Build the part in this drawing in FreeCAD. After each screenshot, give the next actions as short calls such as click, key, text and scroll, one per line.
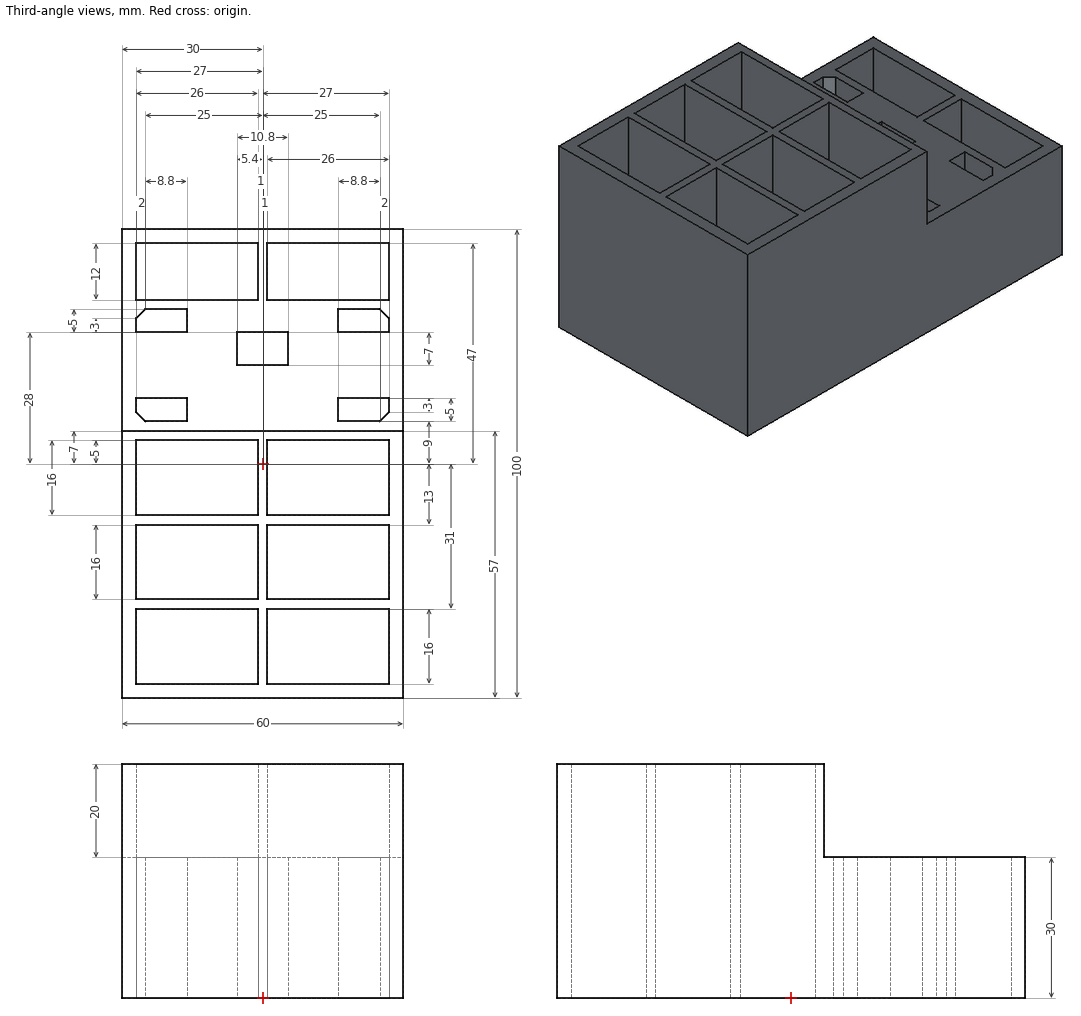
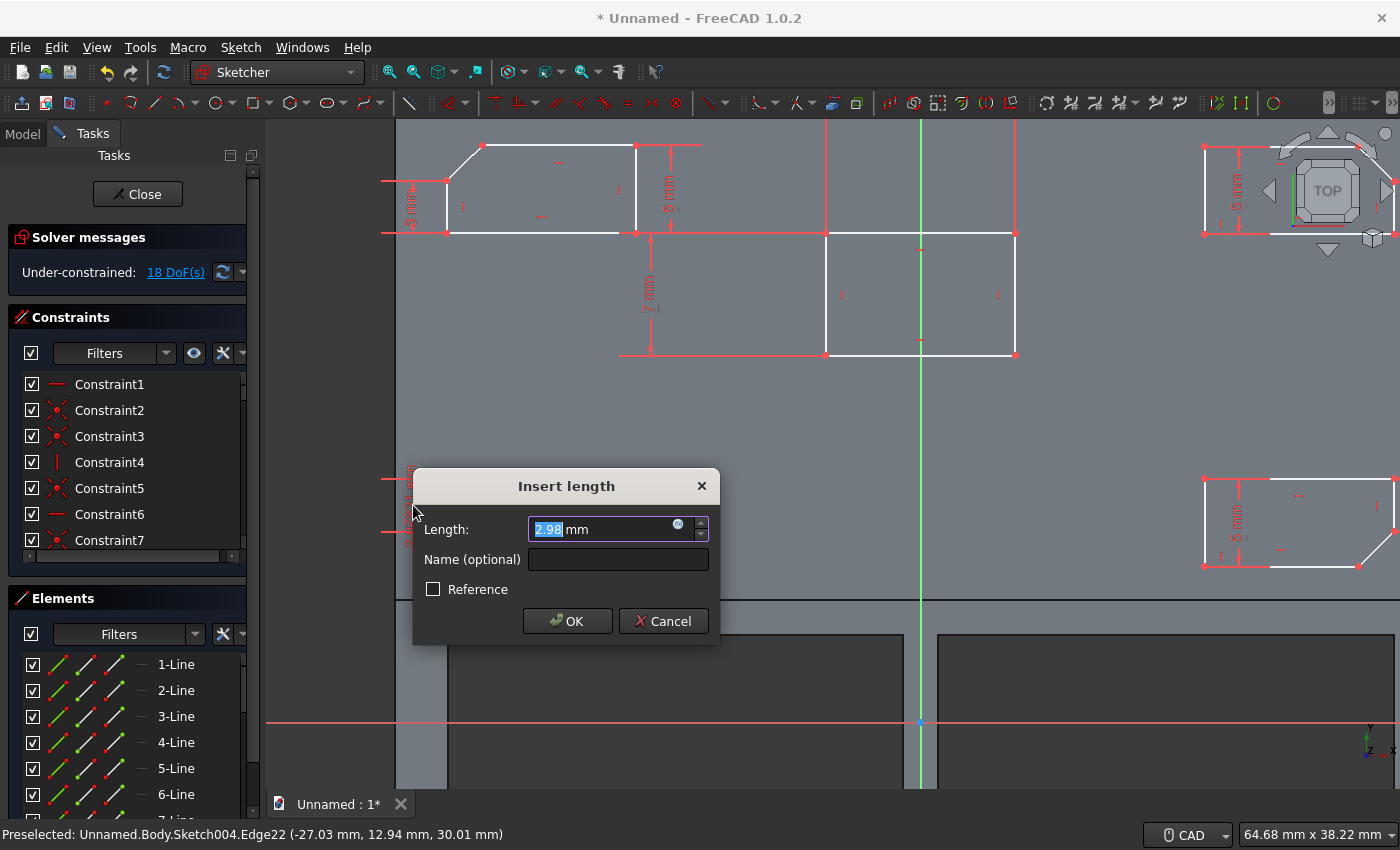
text(3)
key(Return)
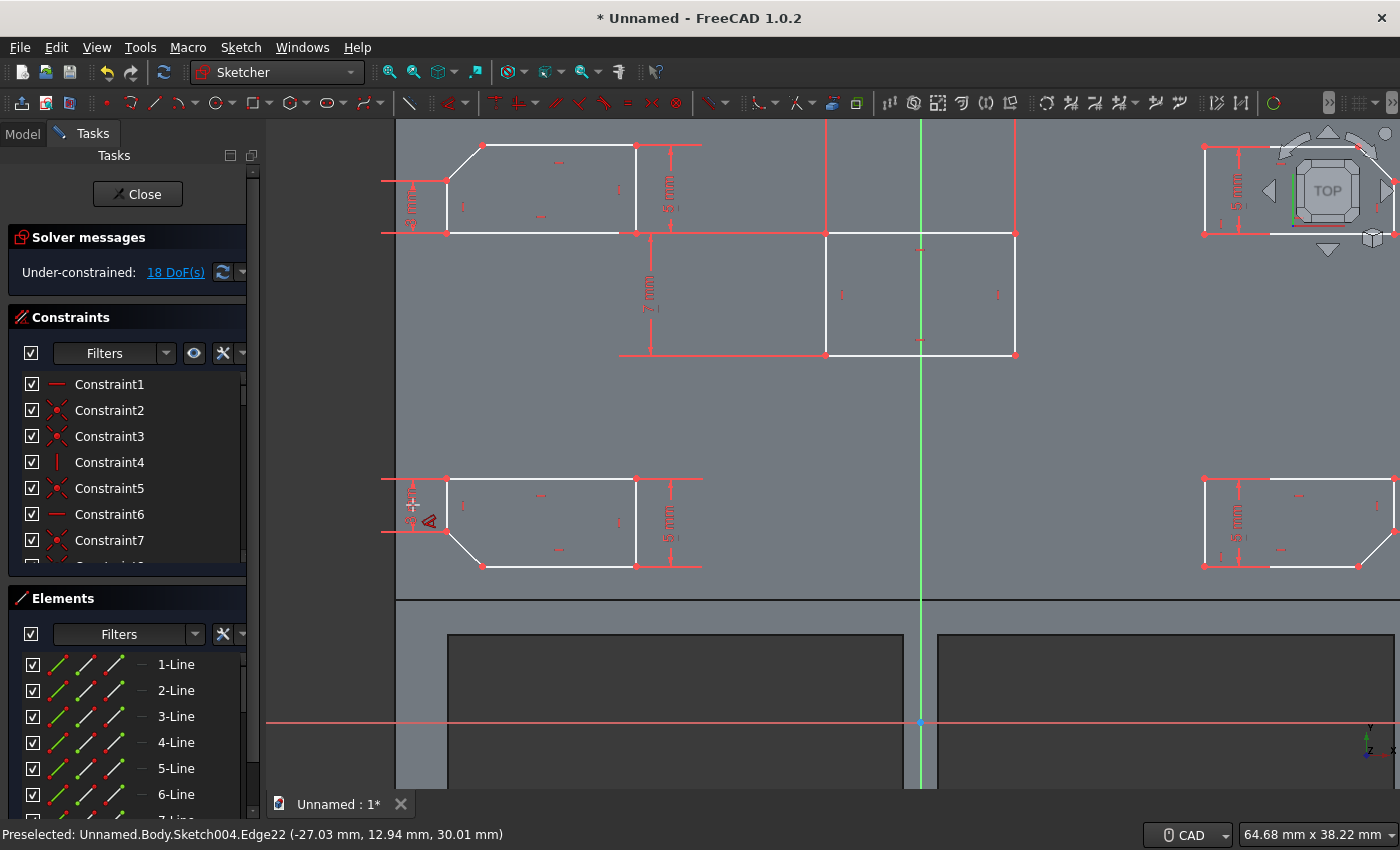
click(1205, 567)
click(887, 645)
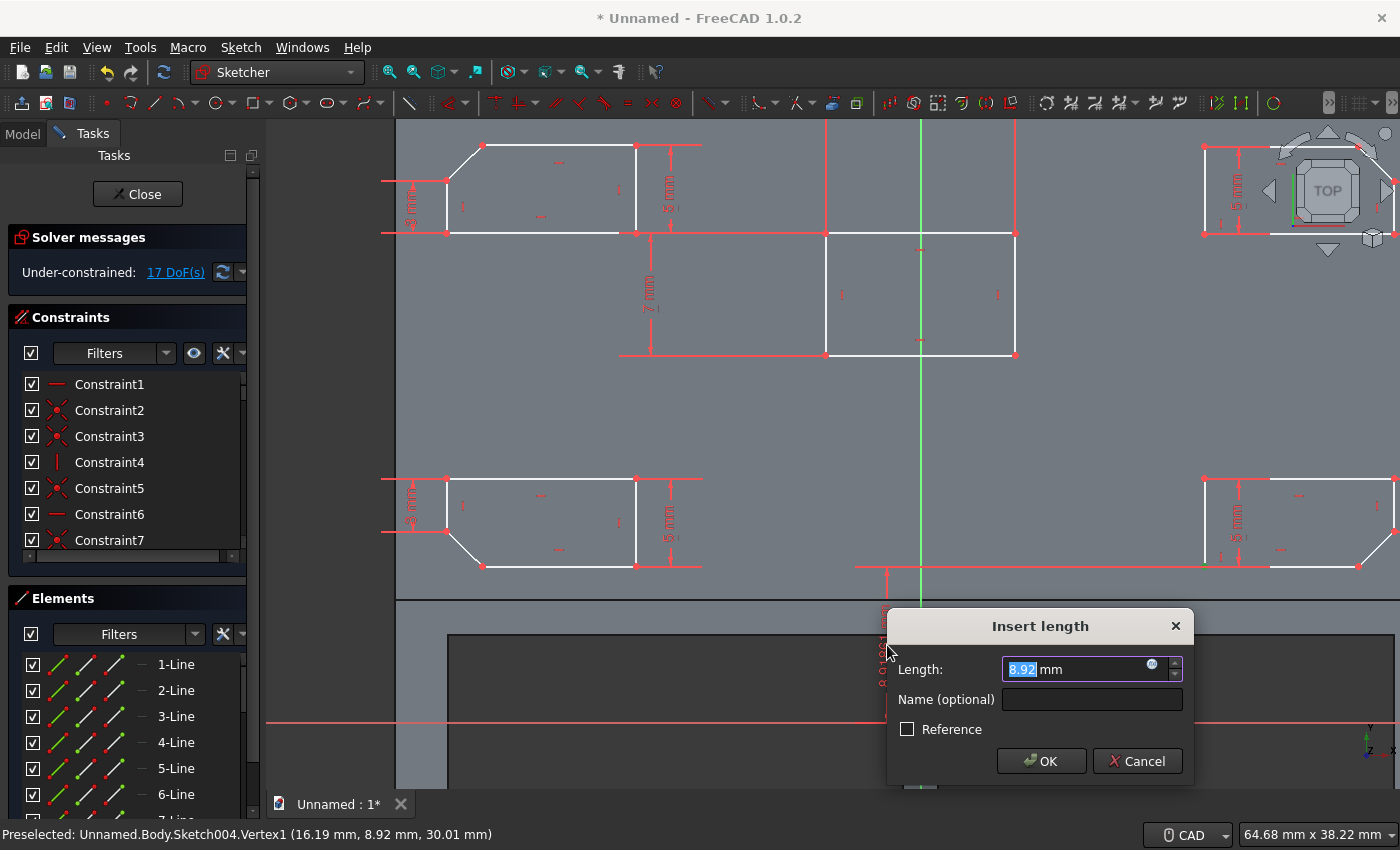
text(9)
key(Return)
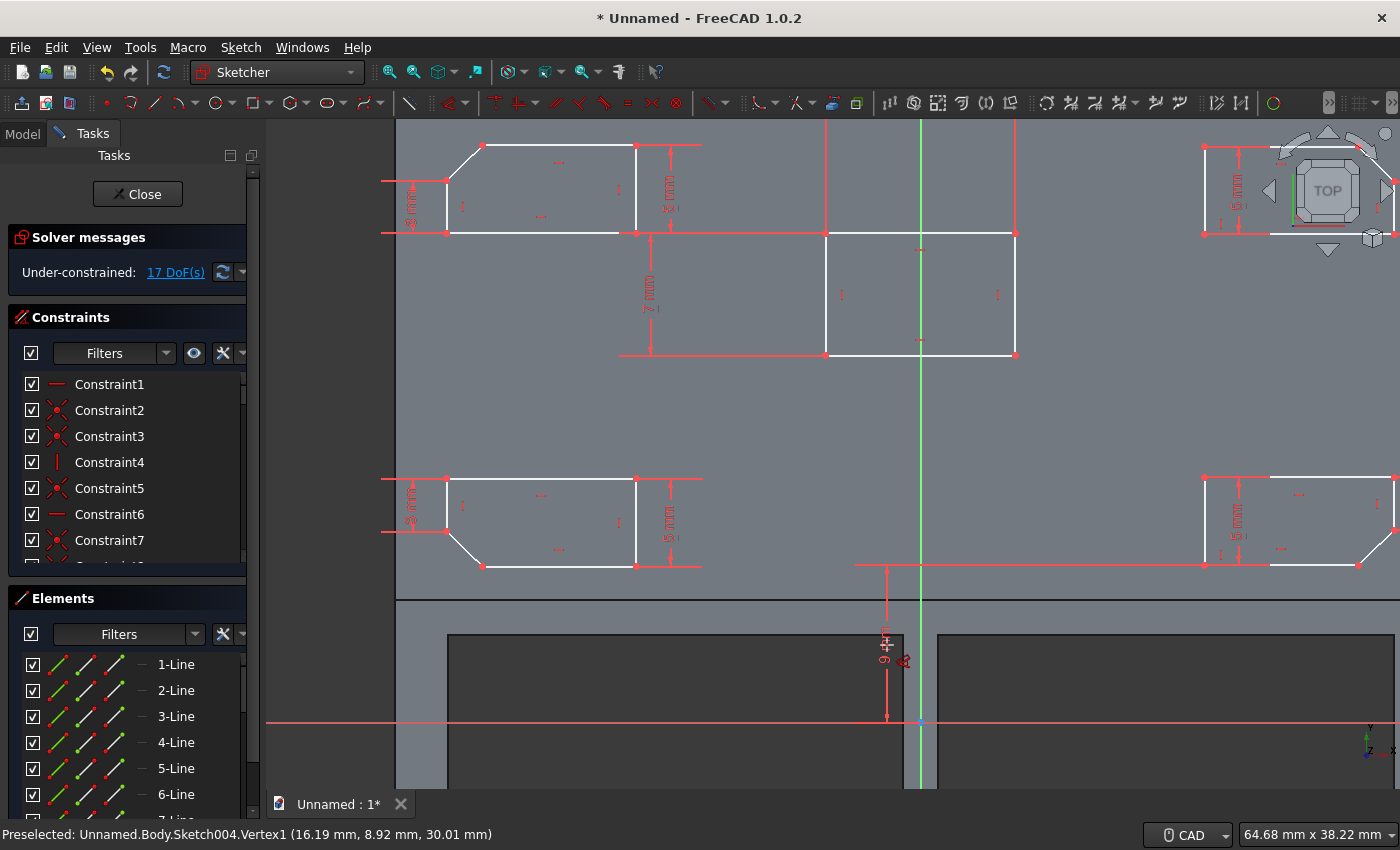
click(636, 567)
click(602, 645)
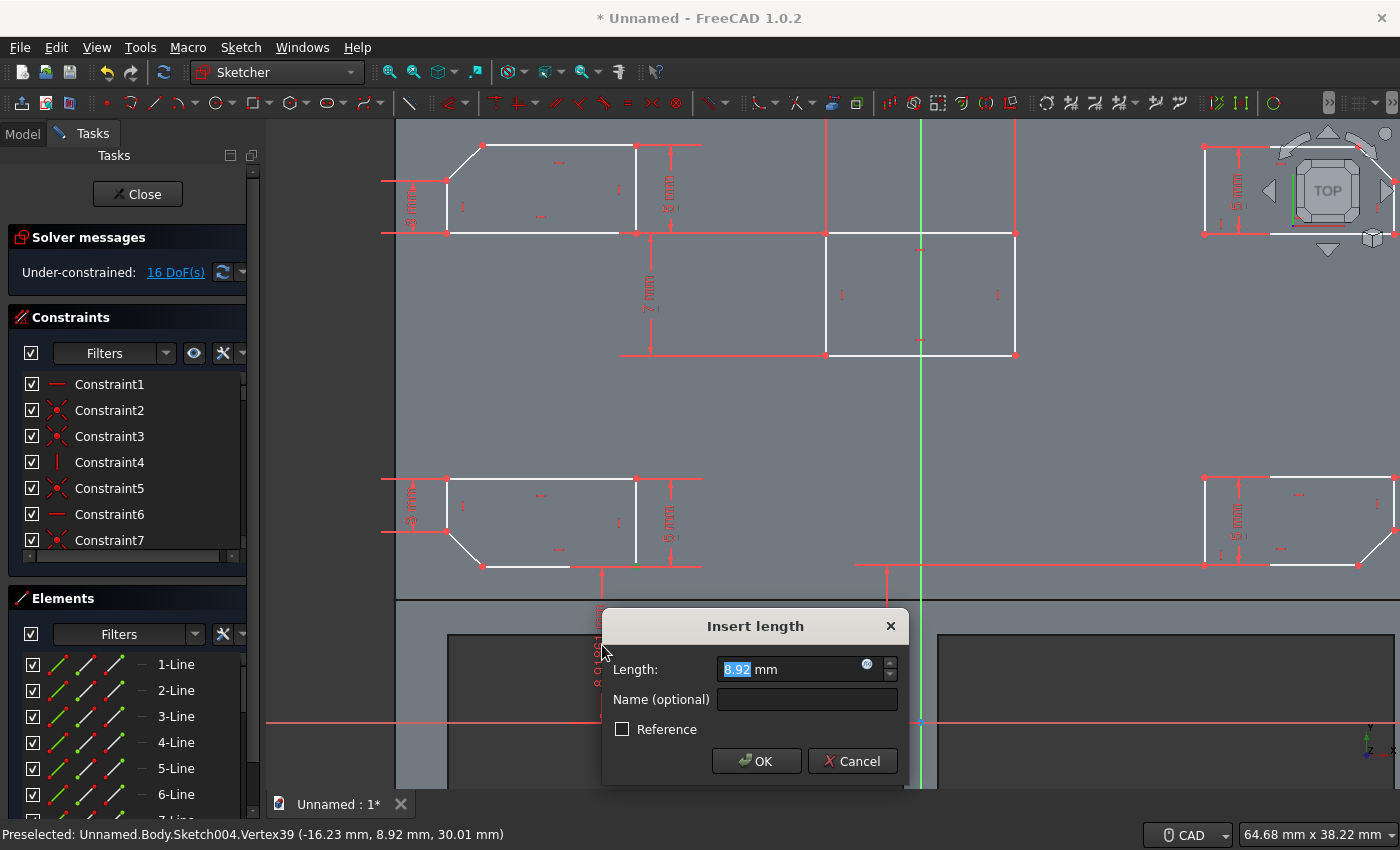
text(9)
key(Return)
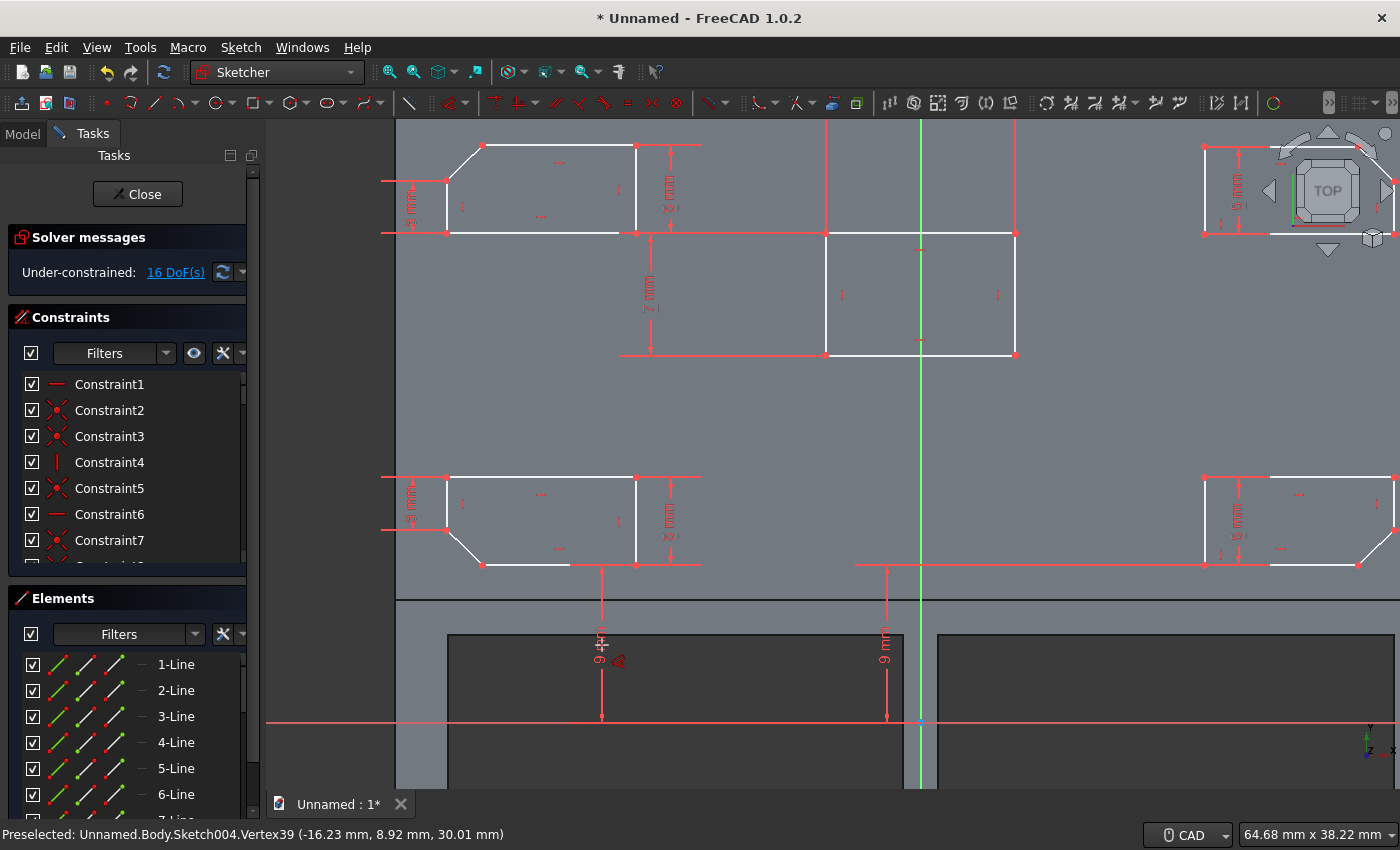
scroll(447, 495, down, 2)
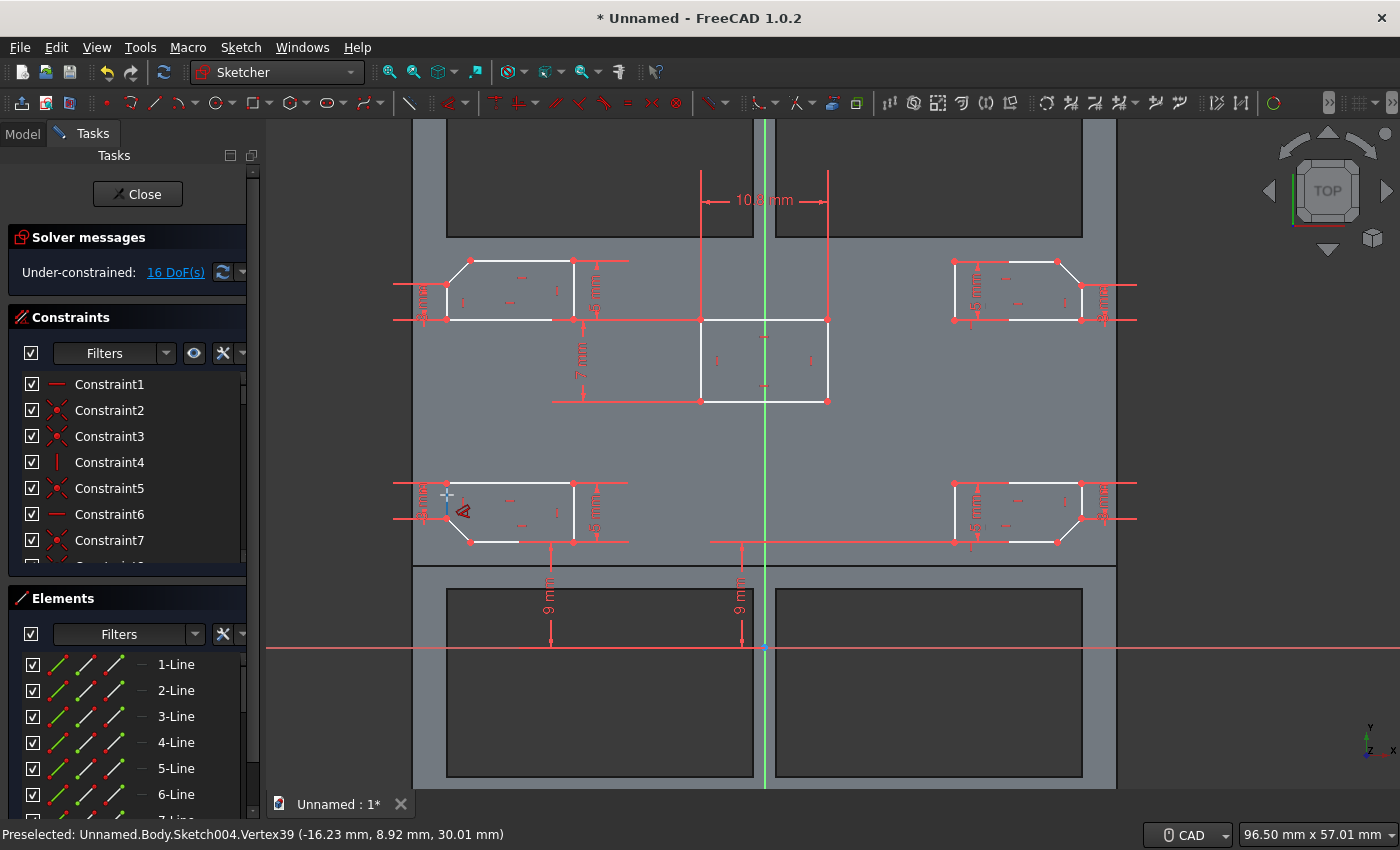
scroll(1065, 535, up, 3)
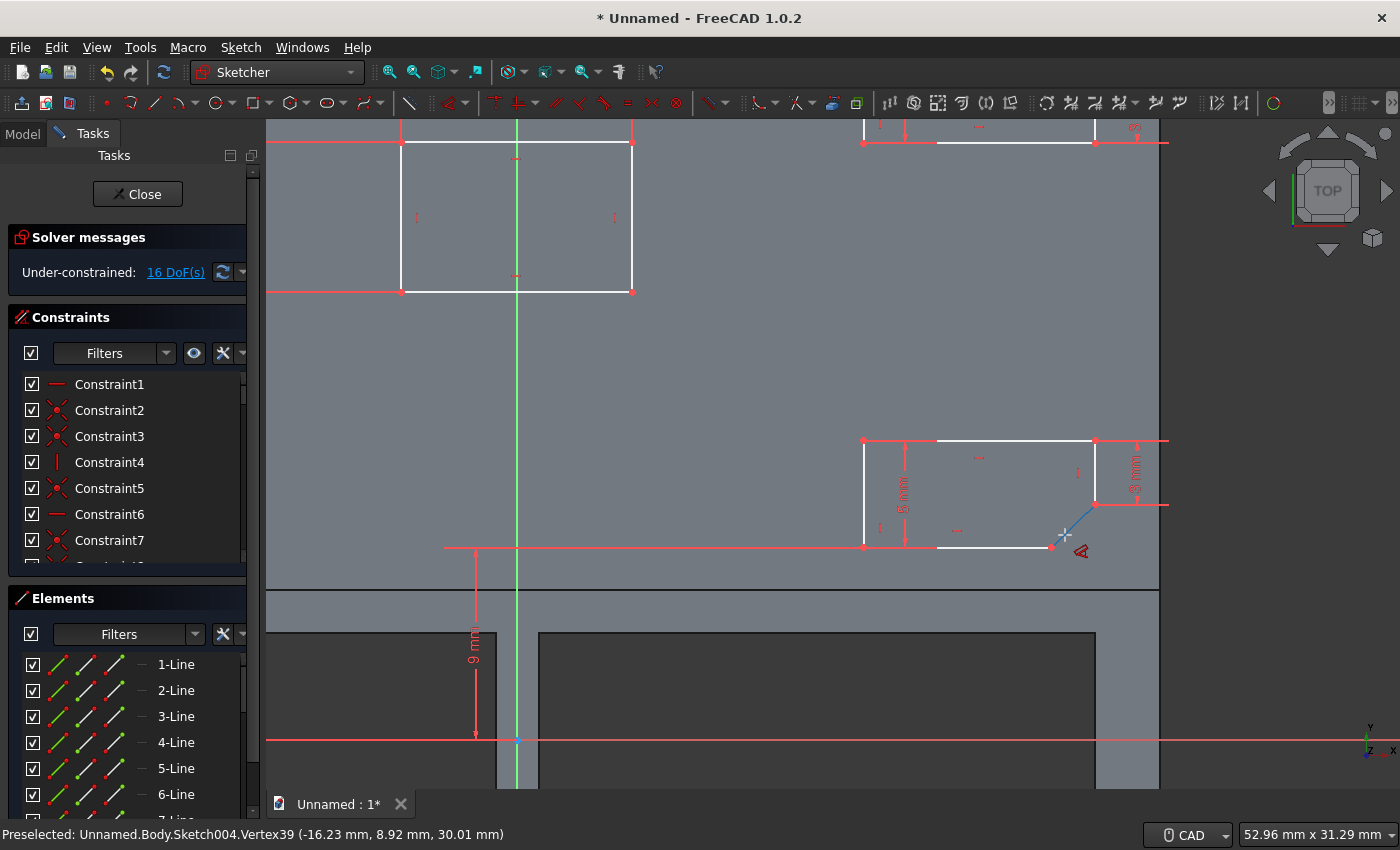
click(1065, 535)
click(1074, 582)